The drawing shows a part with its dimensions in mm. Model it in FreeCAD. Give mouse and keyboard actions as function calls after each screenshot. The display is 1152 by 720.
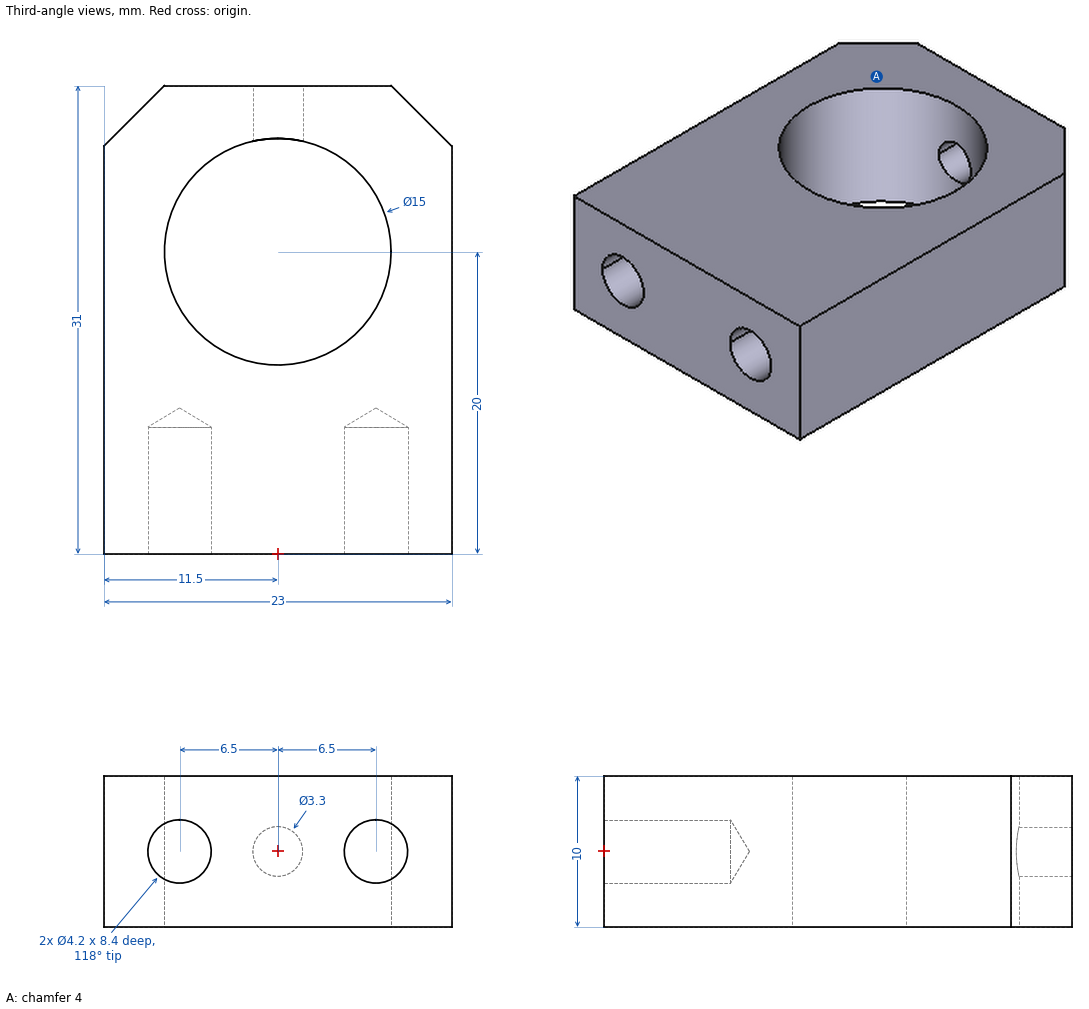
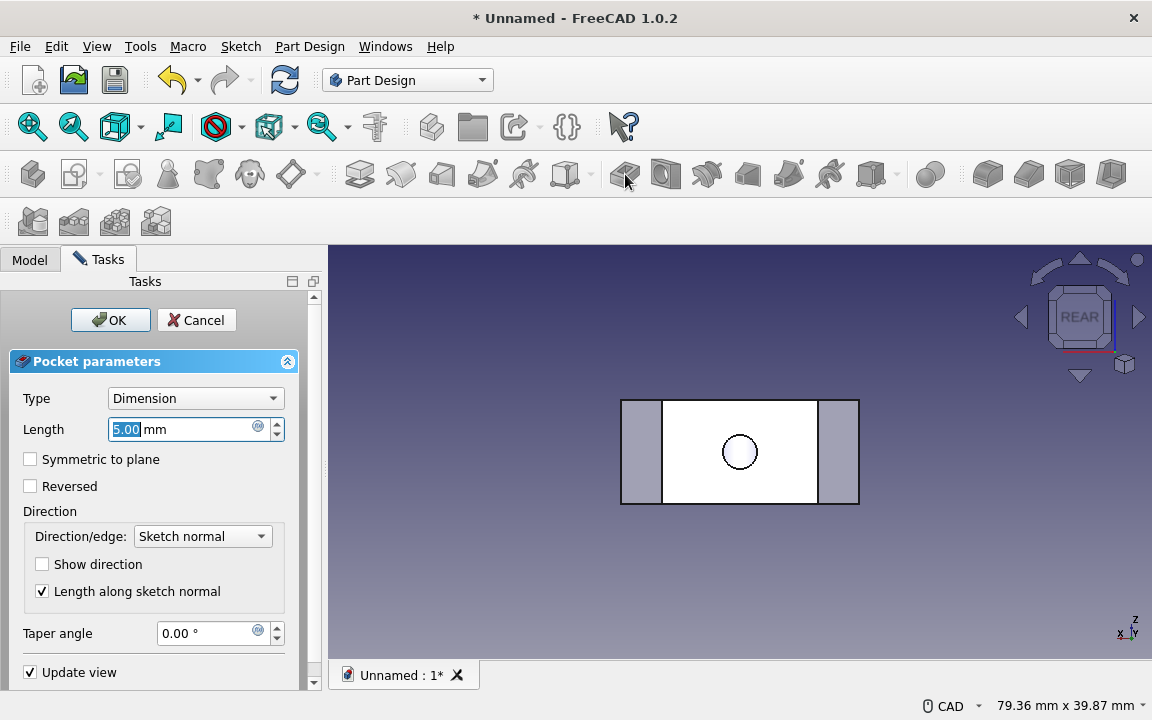
click(196, 398)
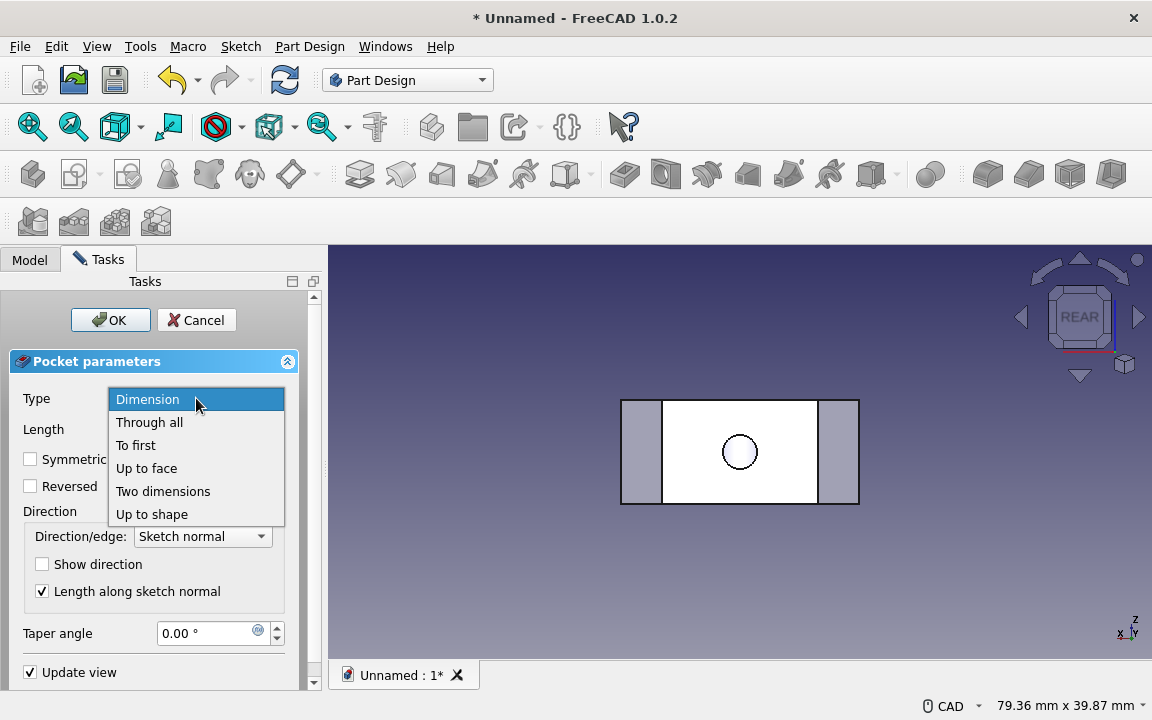
click(194, 446)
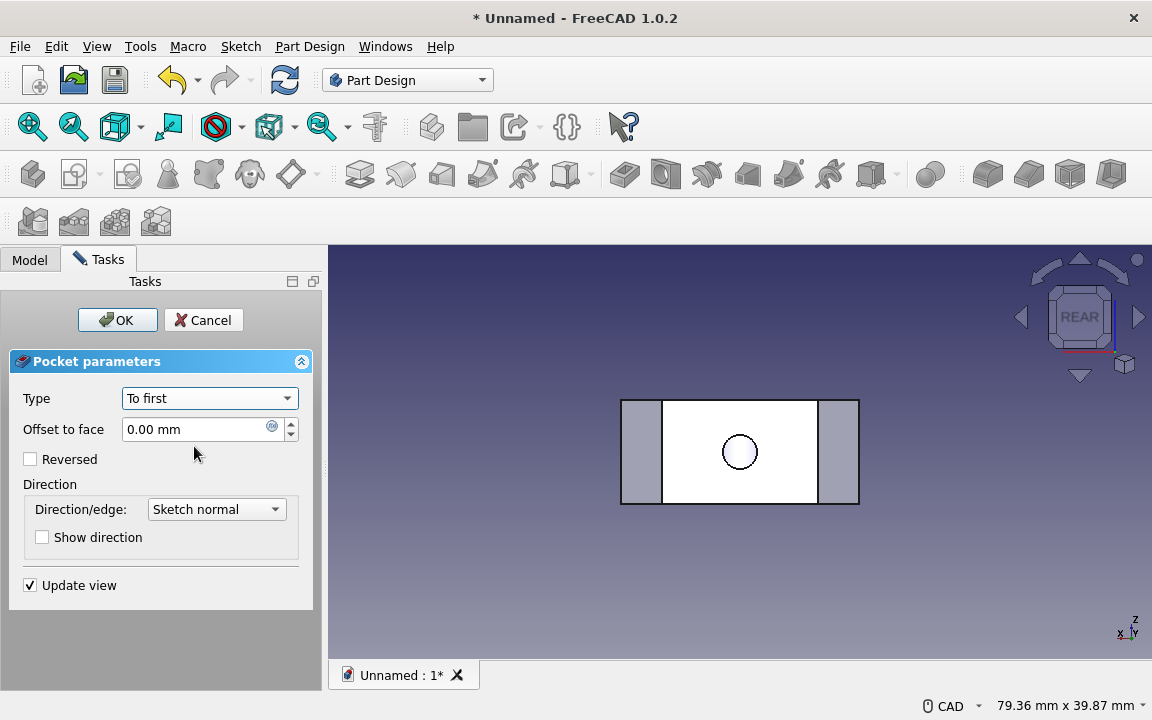
click(118, 320)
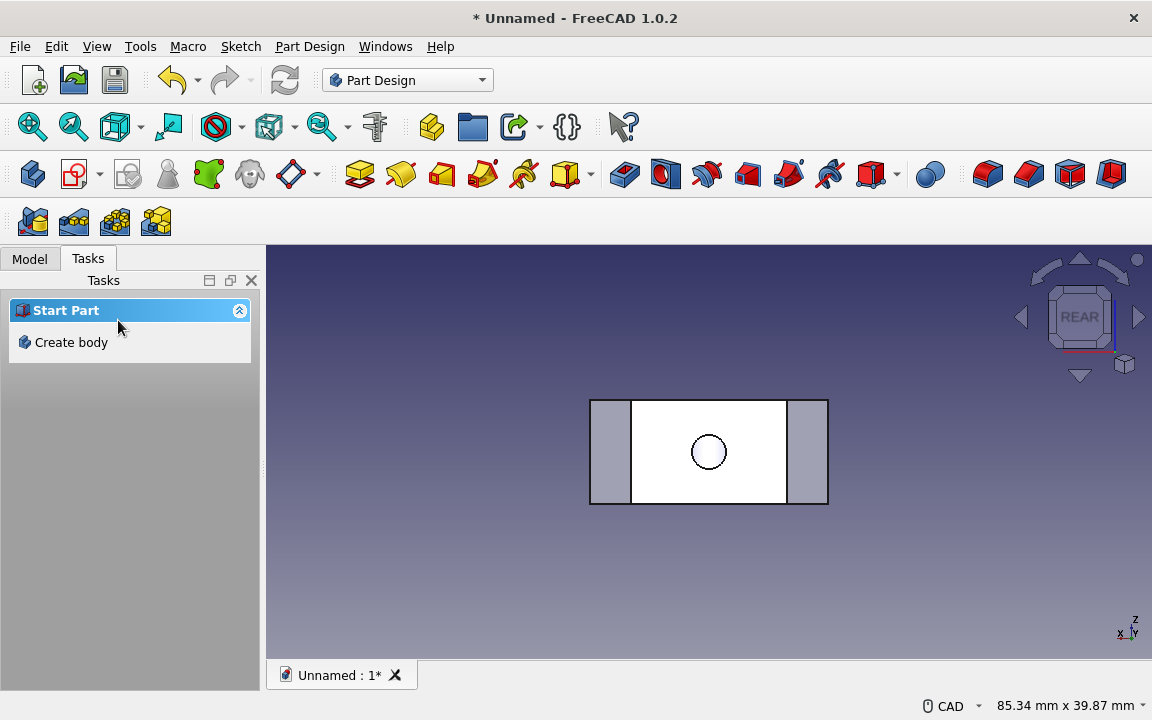
key(v)
key(f)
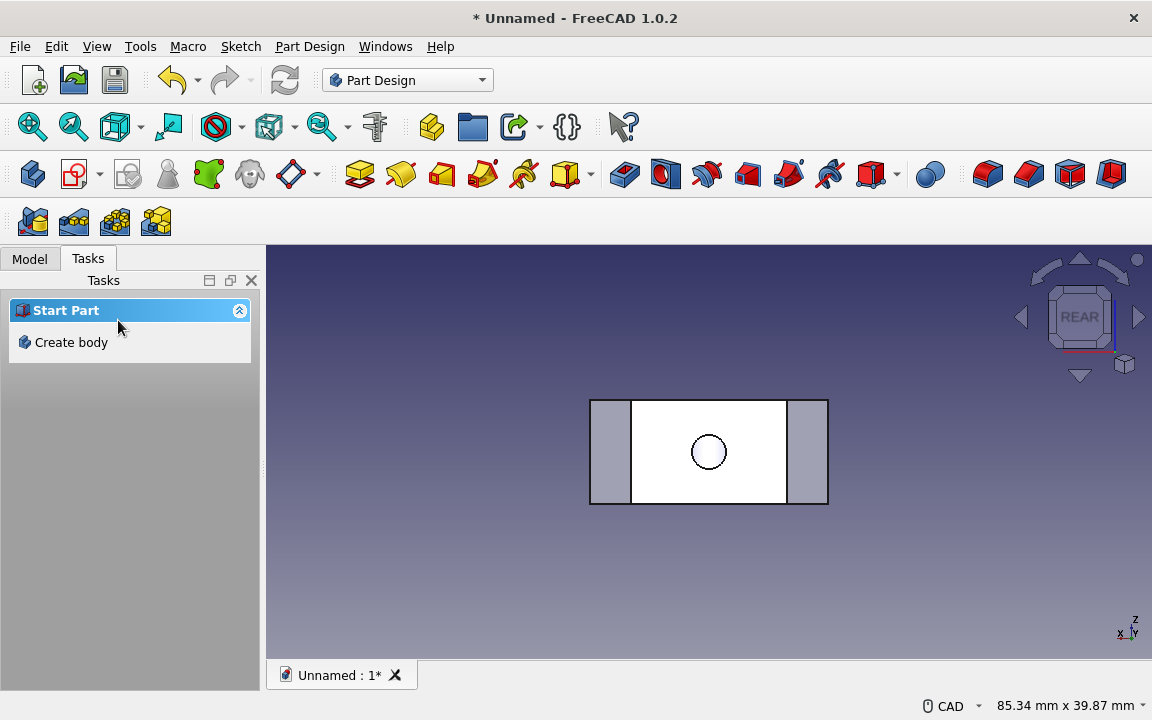
click(74, 174)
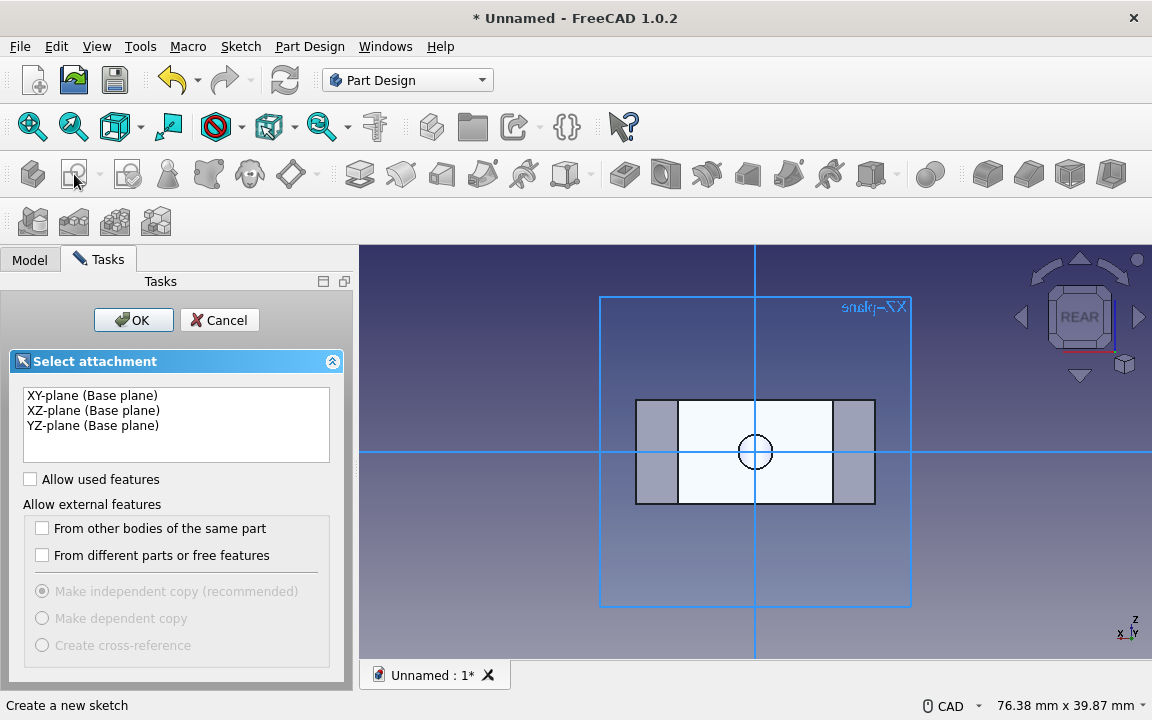
click(84, 410)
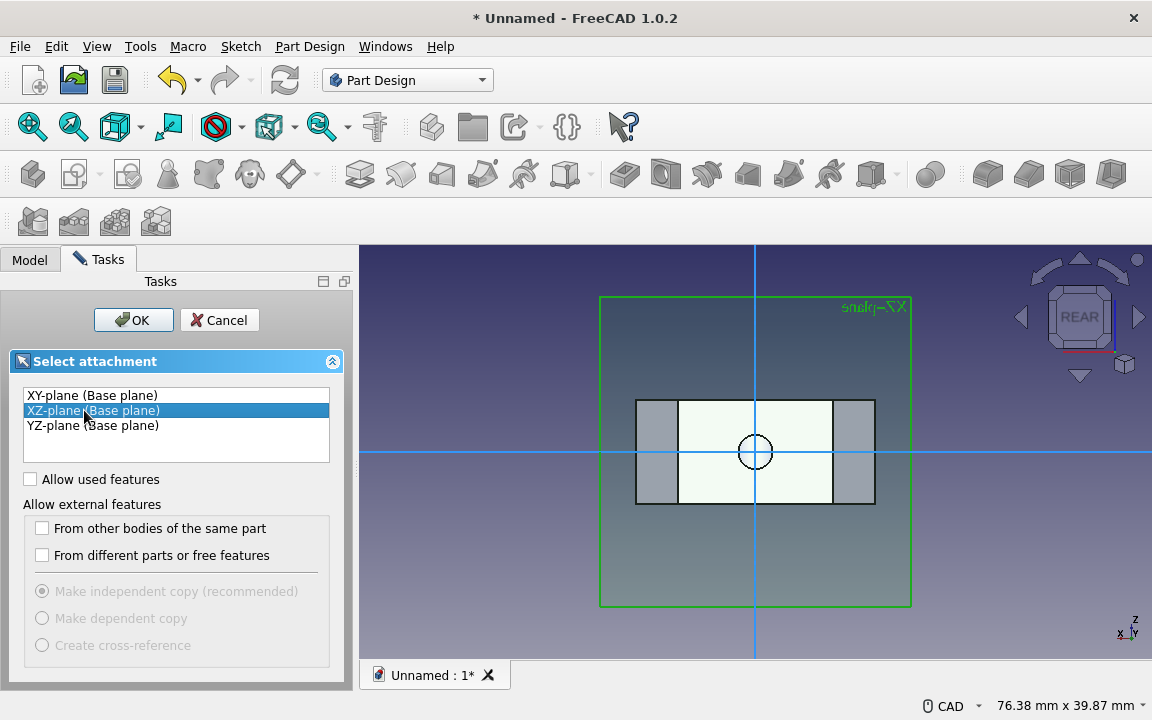
click(134, 320)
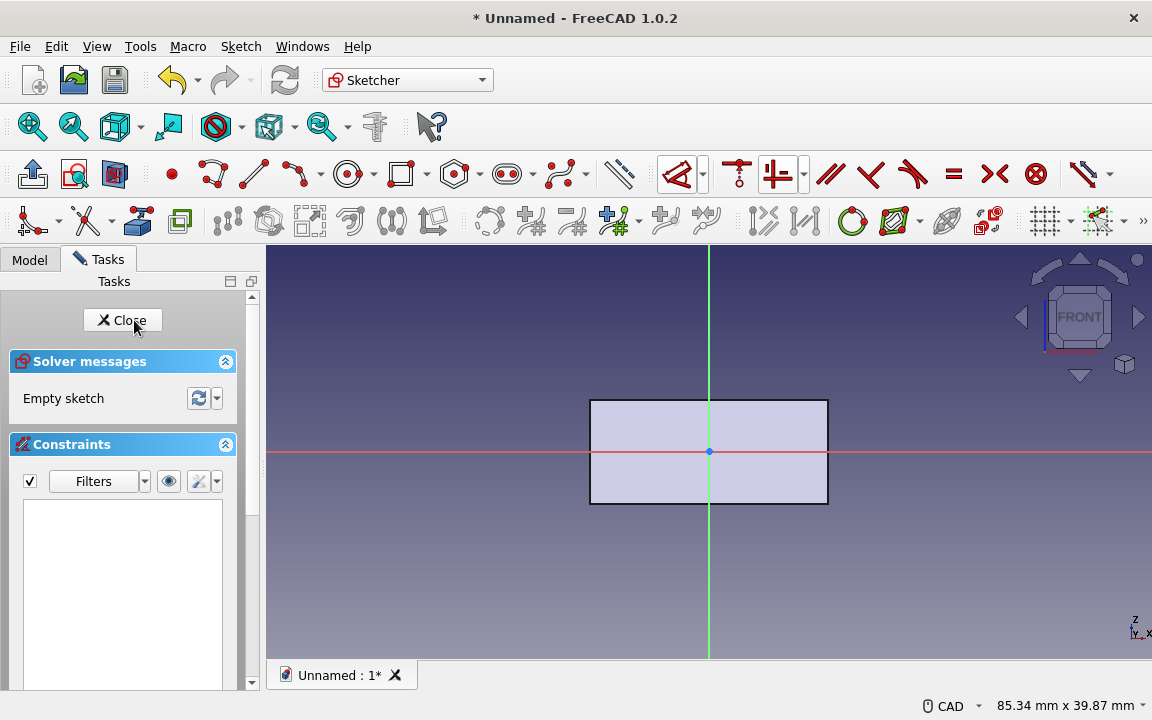
scroll(749, 452, up, 5)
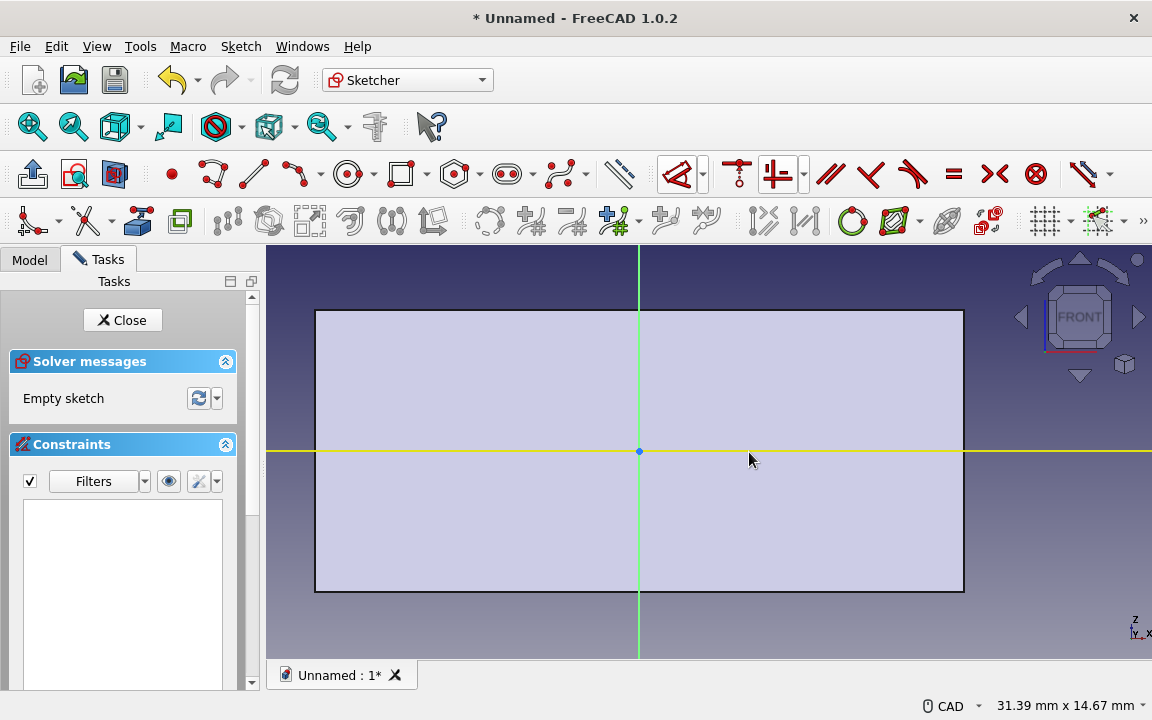
click(348, 174)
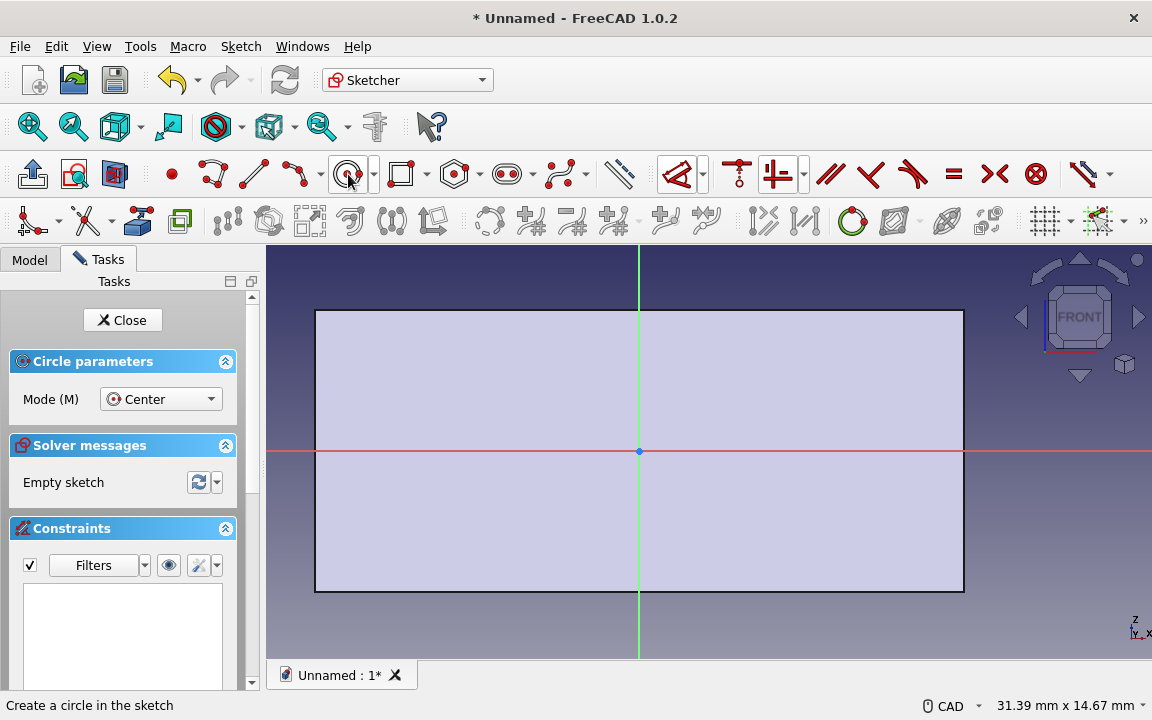
click(456, 451)
move(498, 409)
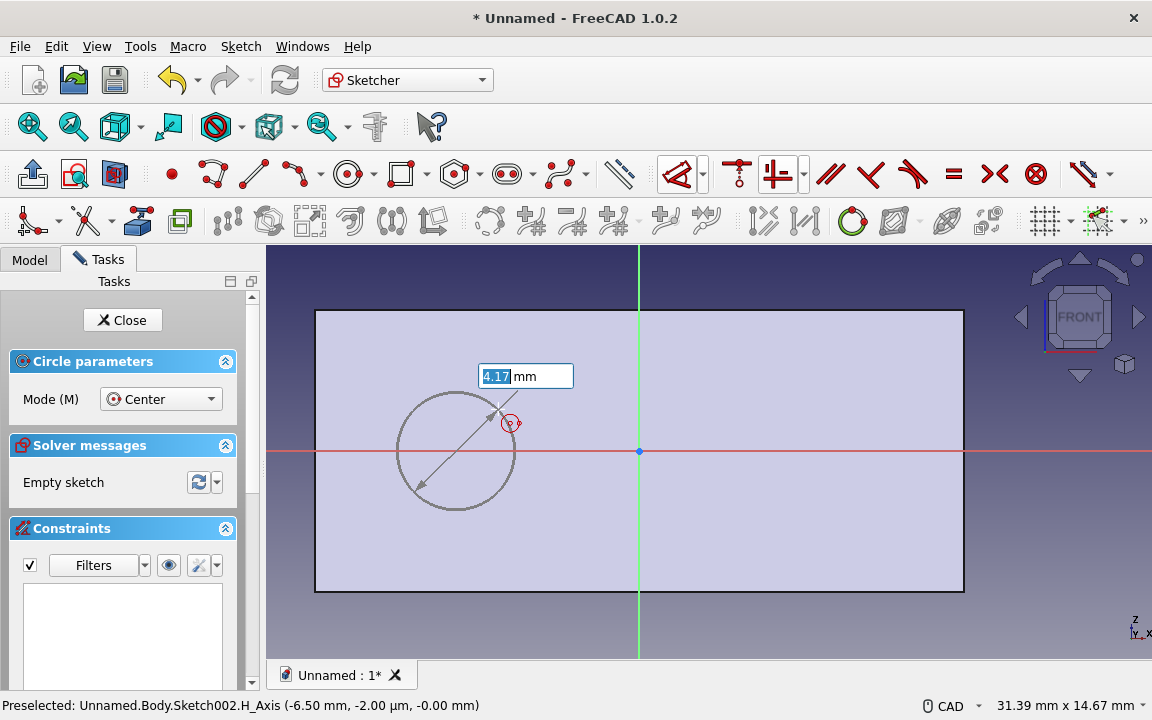
text(4.2)
key(Return)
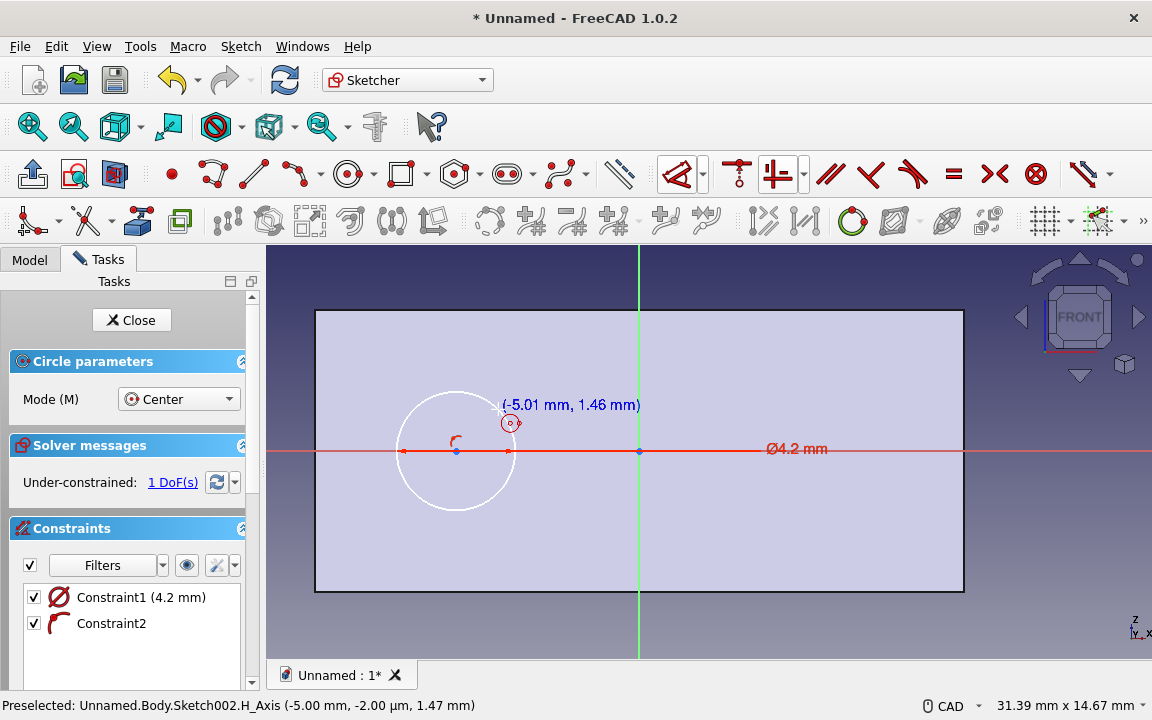
click(823, 451)
move(865, 409)